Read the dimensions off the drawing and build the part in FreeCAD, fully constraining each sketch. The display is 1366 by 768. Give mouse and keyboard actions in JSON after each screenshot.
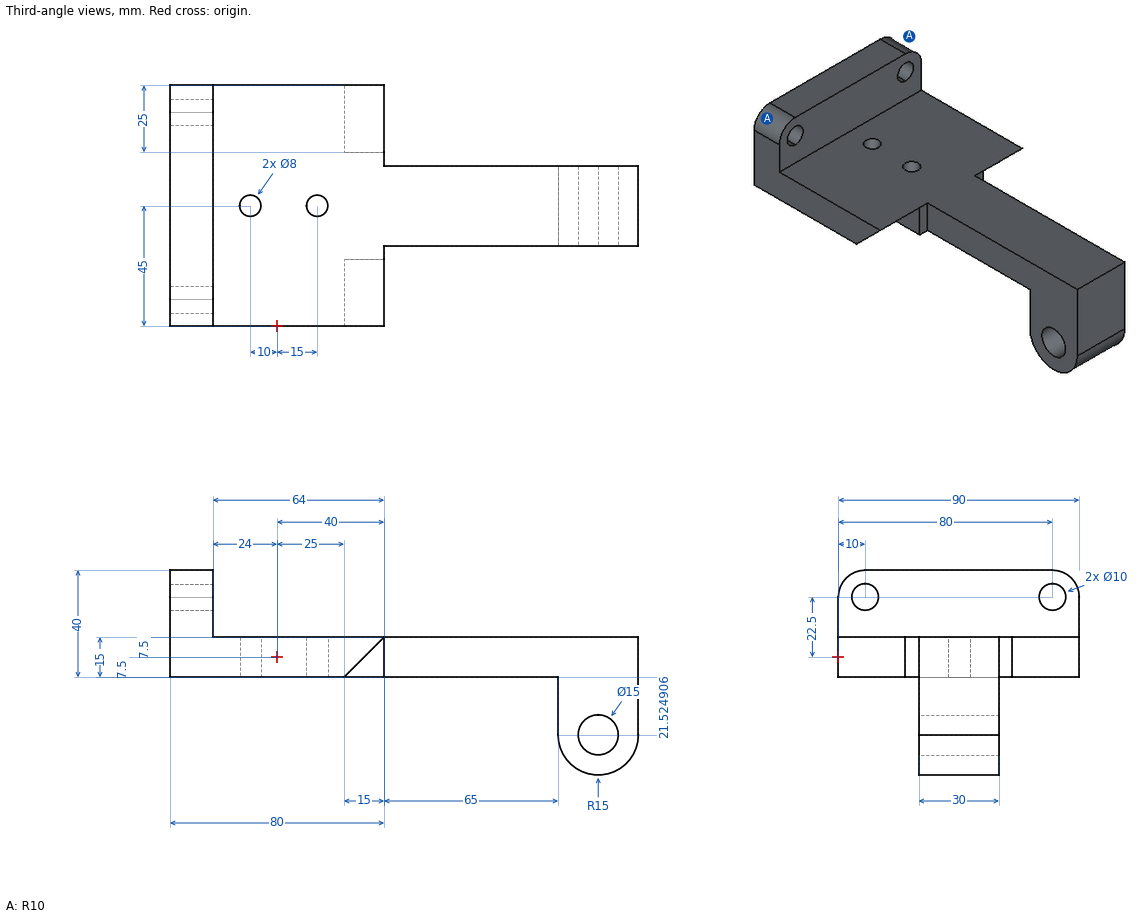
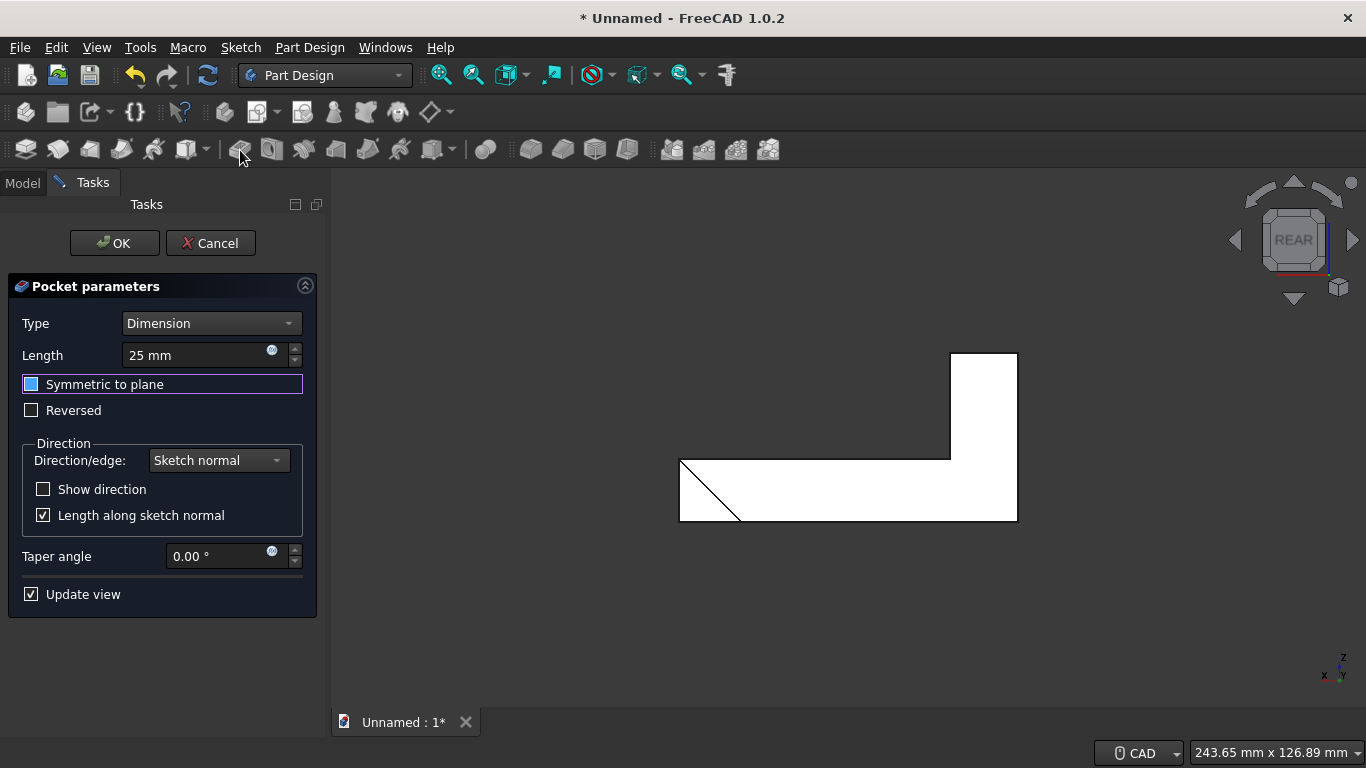
{"action": "left_click", "coordinate": [115, 243]}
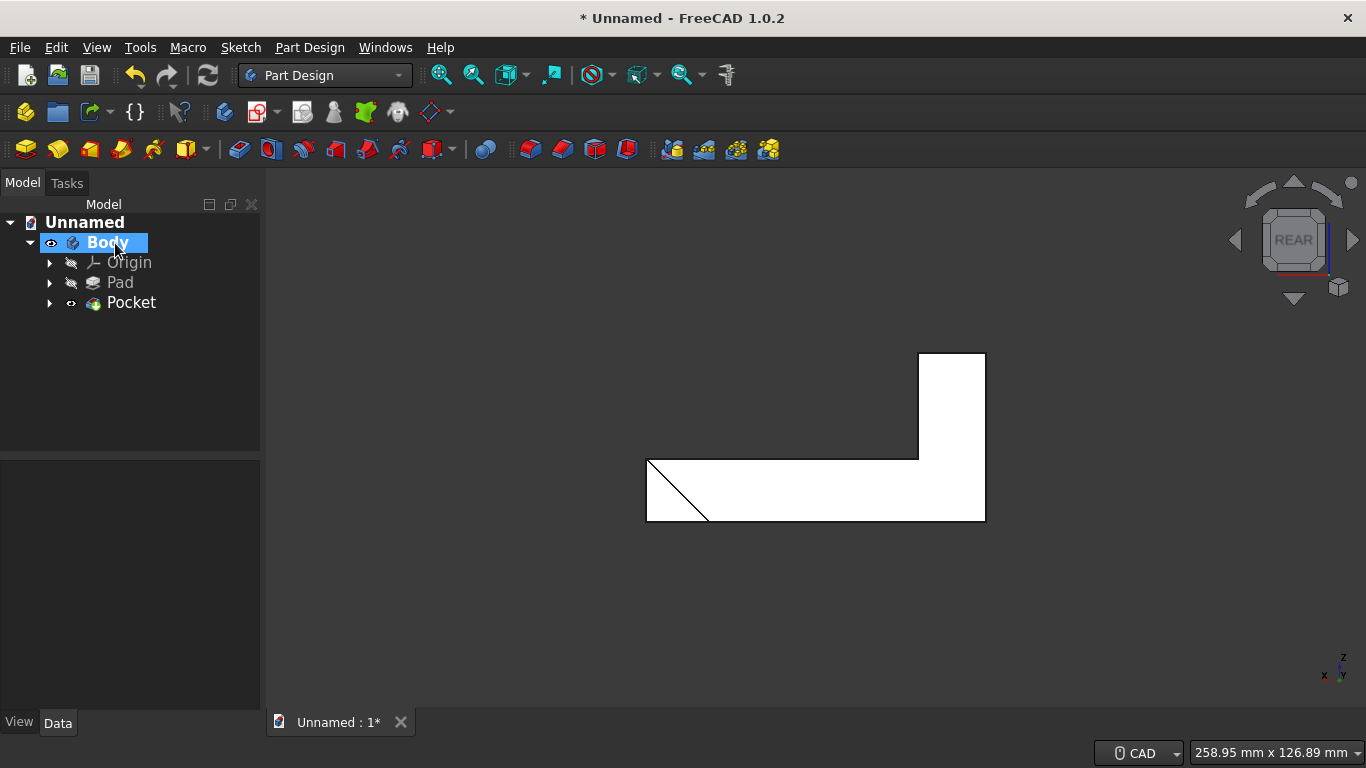
{"action": "left_click", "coordinate": [442, 76]}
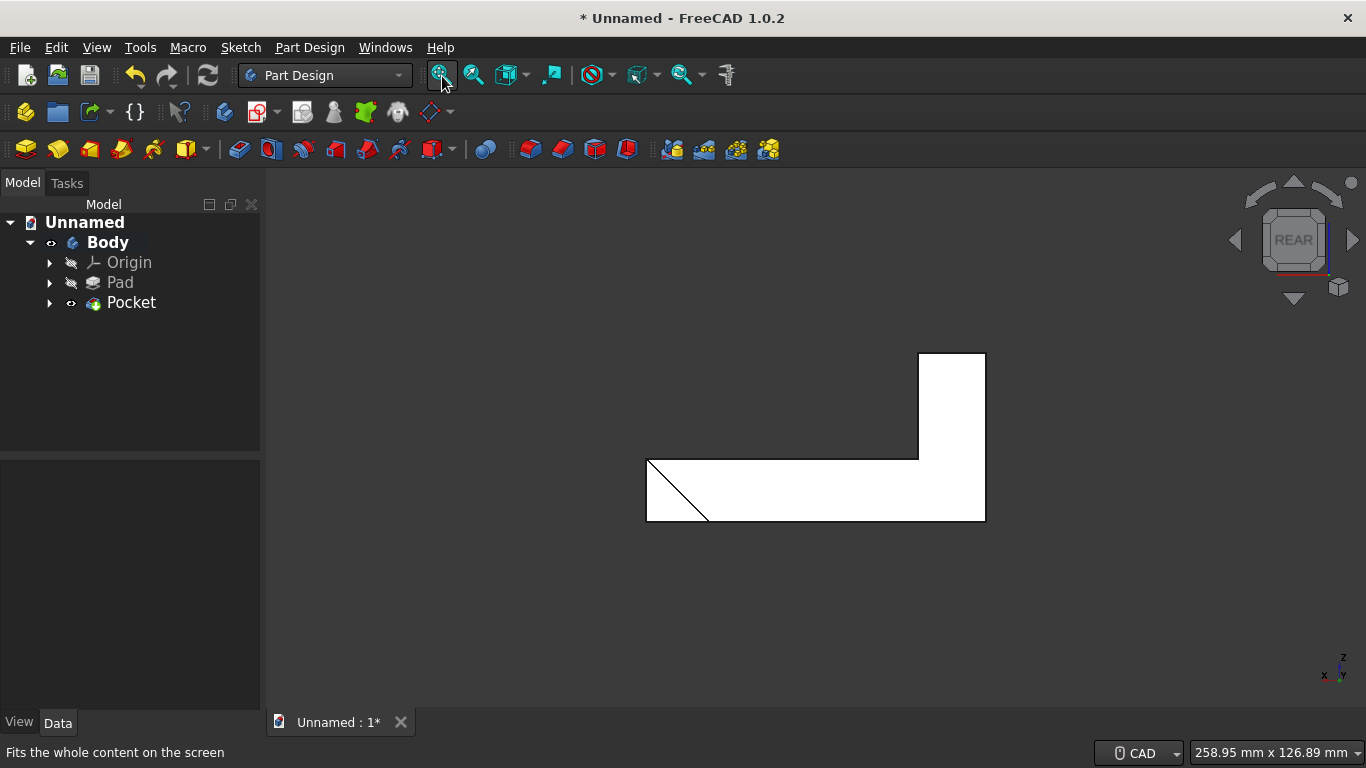
{"action": "left_click", "coordinate": [50, 263]}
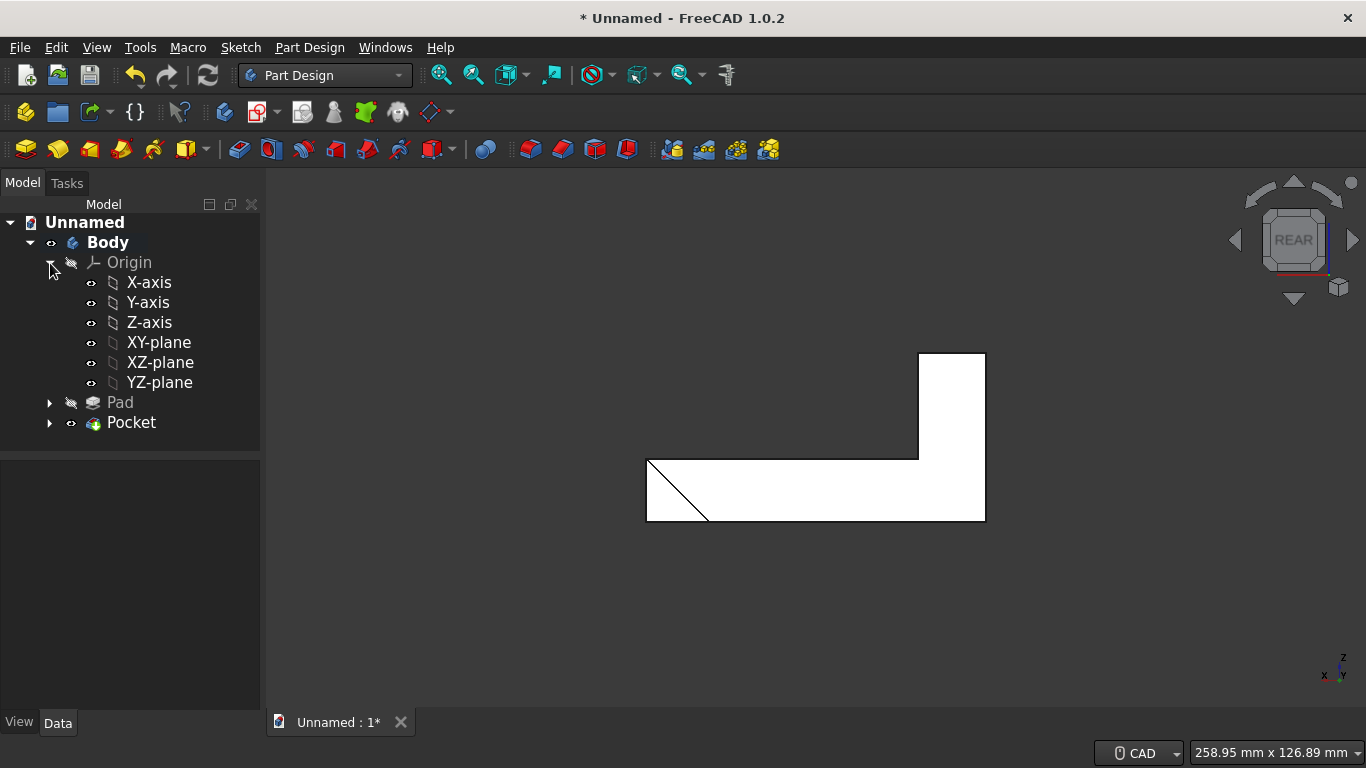
{"action": "left_click", "coordinate": [136, 363]}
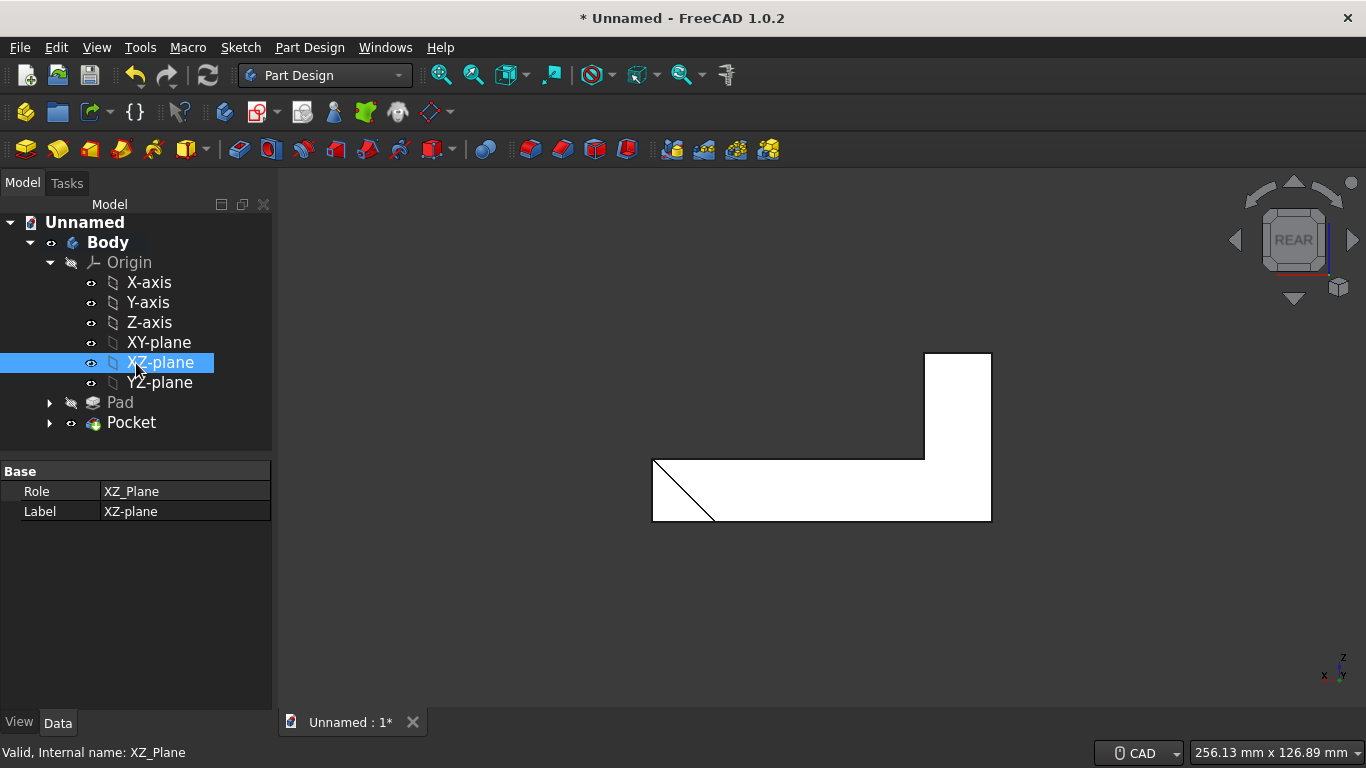
{"action": "left_click", "coordinate": [430, 112]}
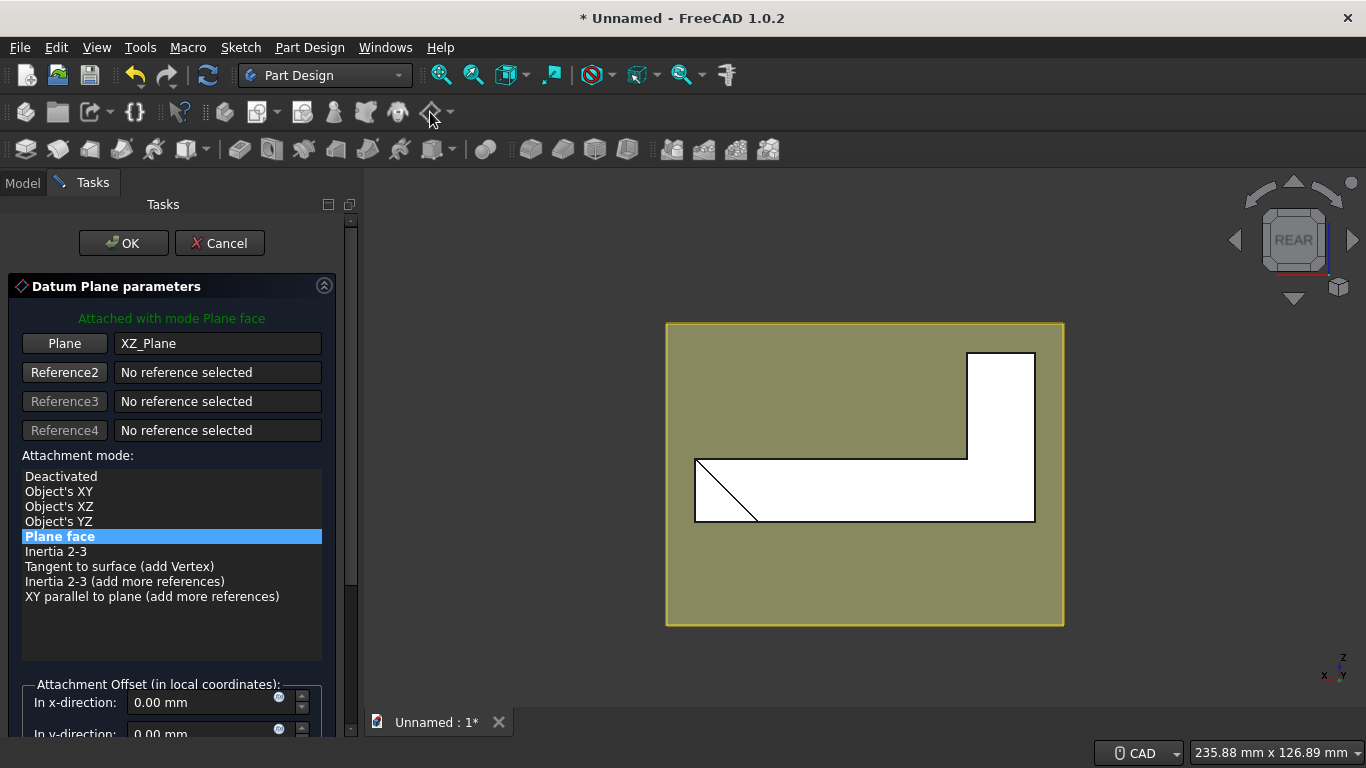
{"action": "scroll", "coordinate": [351, 475], "scroll_direction": "down", "scroll_amount": 2}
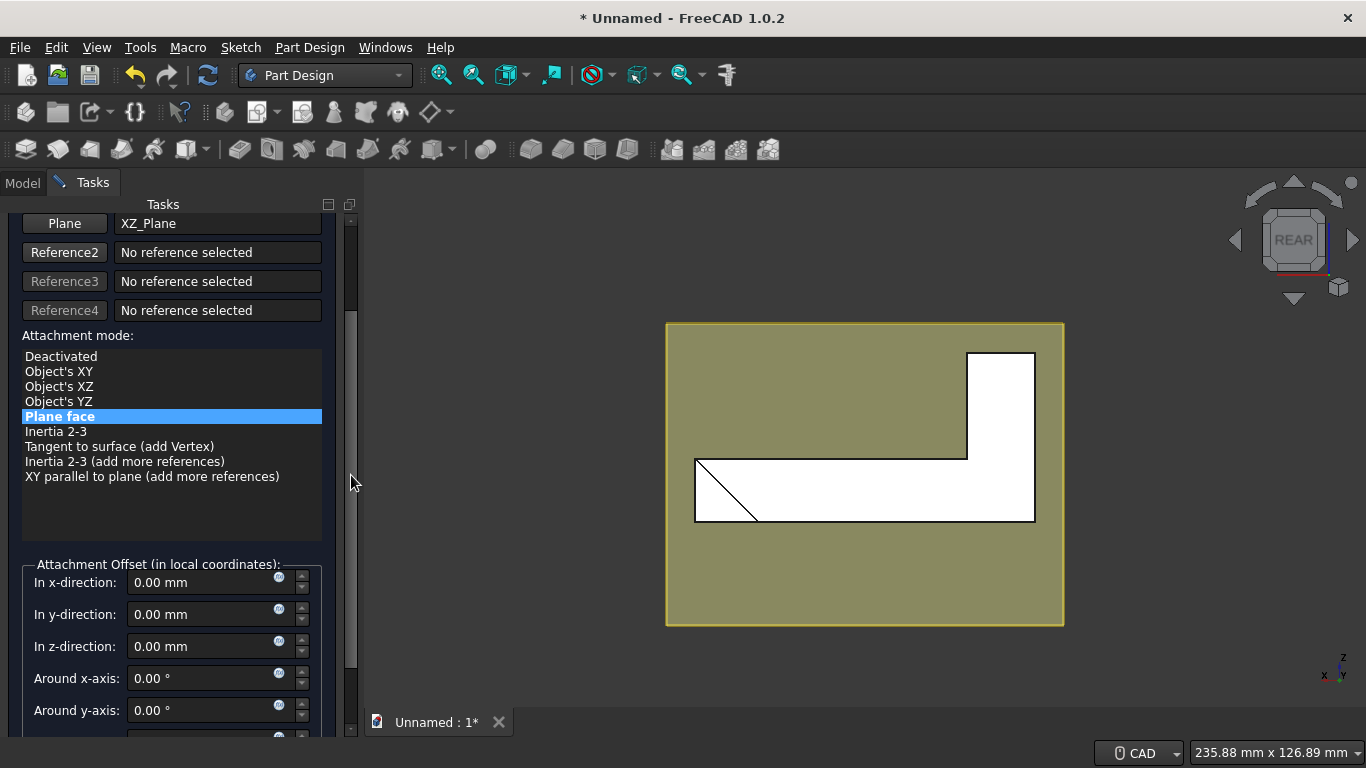
{"action": "triple_click", "coordinate": [210, 646]}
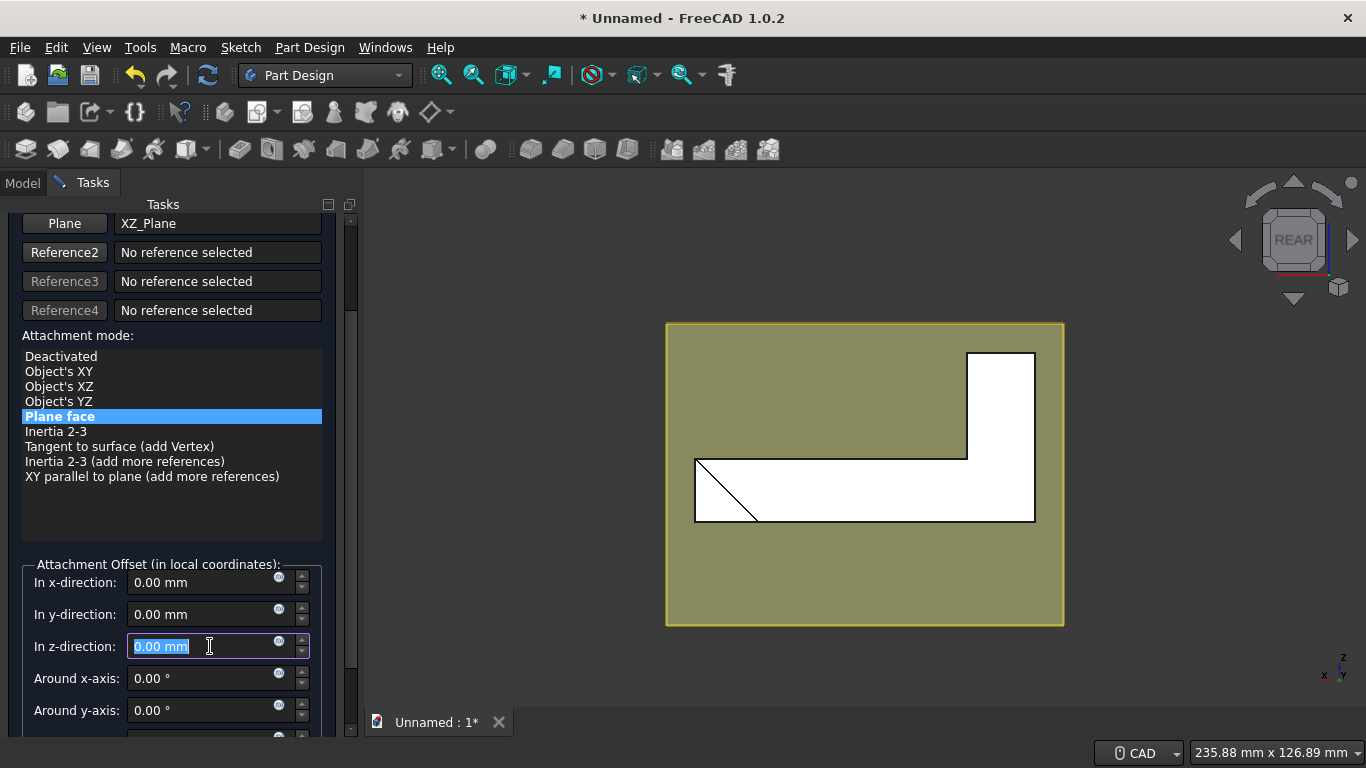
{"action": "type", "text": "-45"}
{"action": "key", "text": "Tab"}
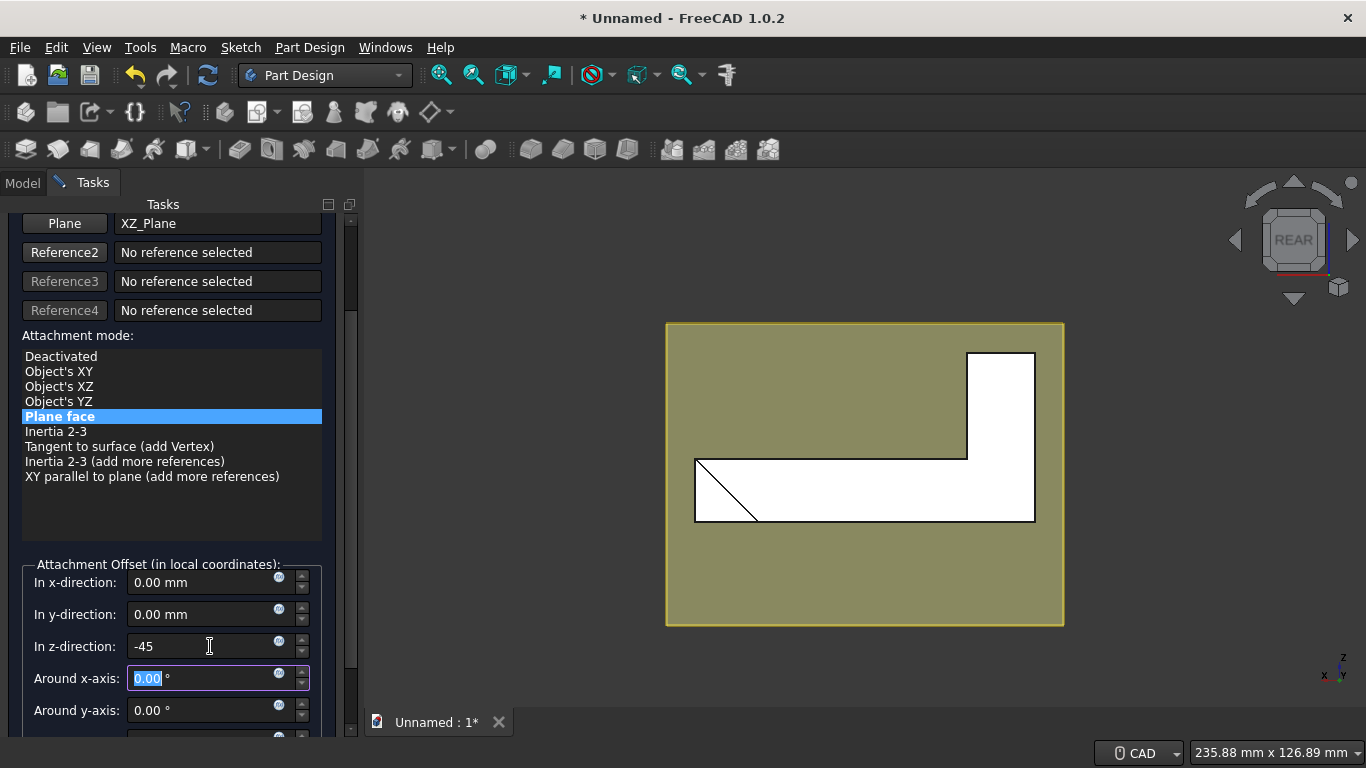
{"action": "scroll", "coordinate": [351, 475], "scroll_direction": "up", "scroll_amount": 3}